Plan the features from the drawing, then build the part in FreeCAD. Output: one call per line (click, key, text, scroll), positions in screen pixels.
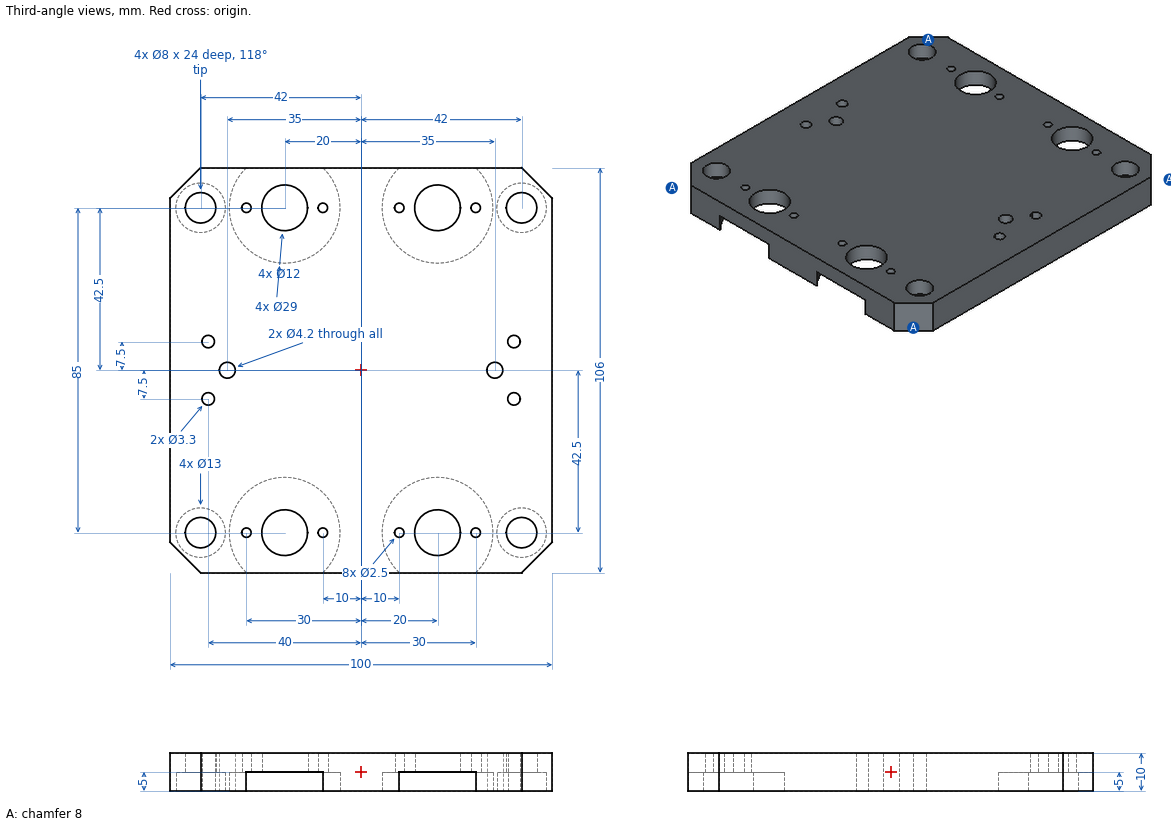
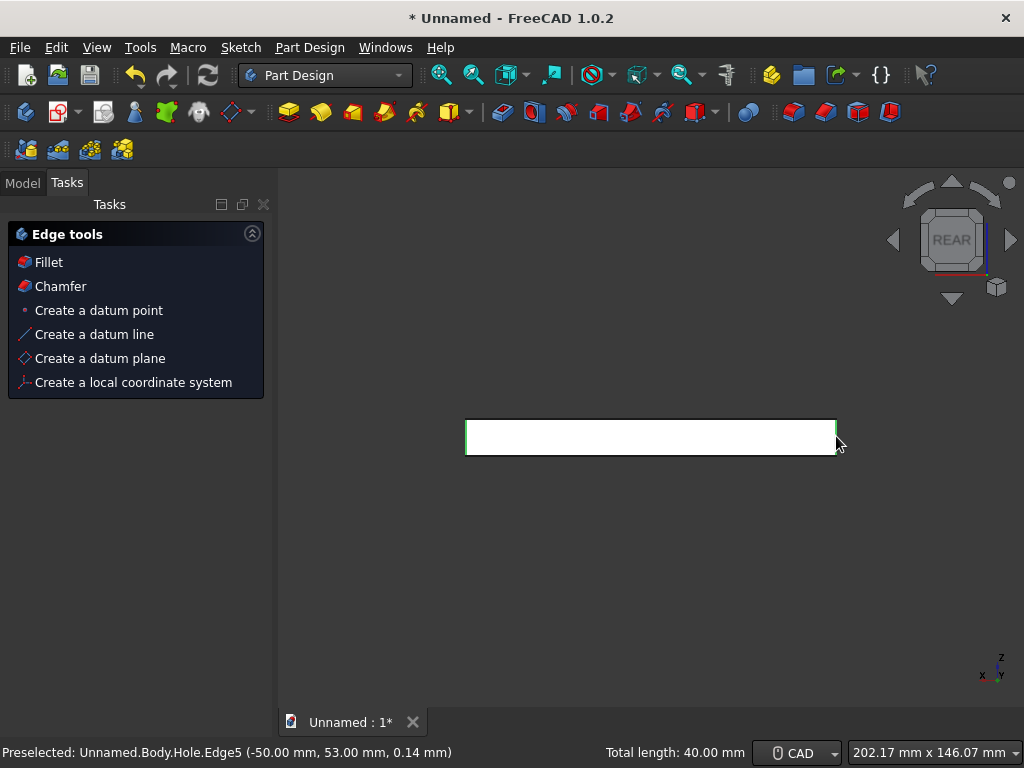
click(826, 112)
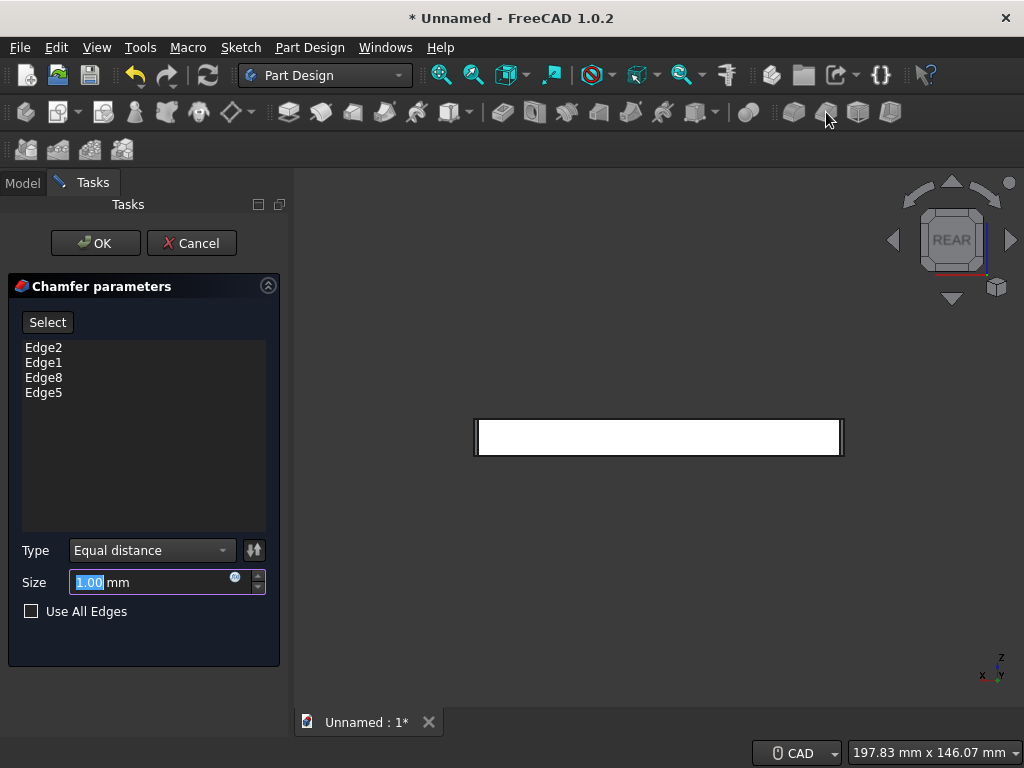
text(8)
key(Tab)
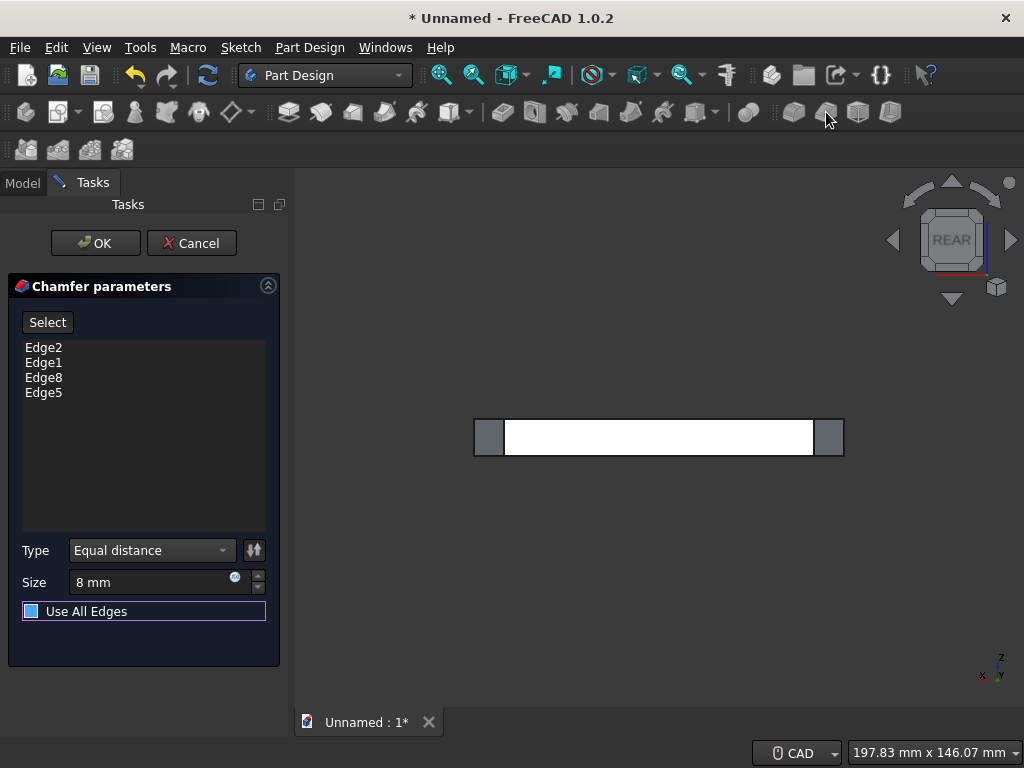
click(96, 243)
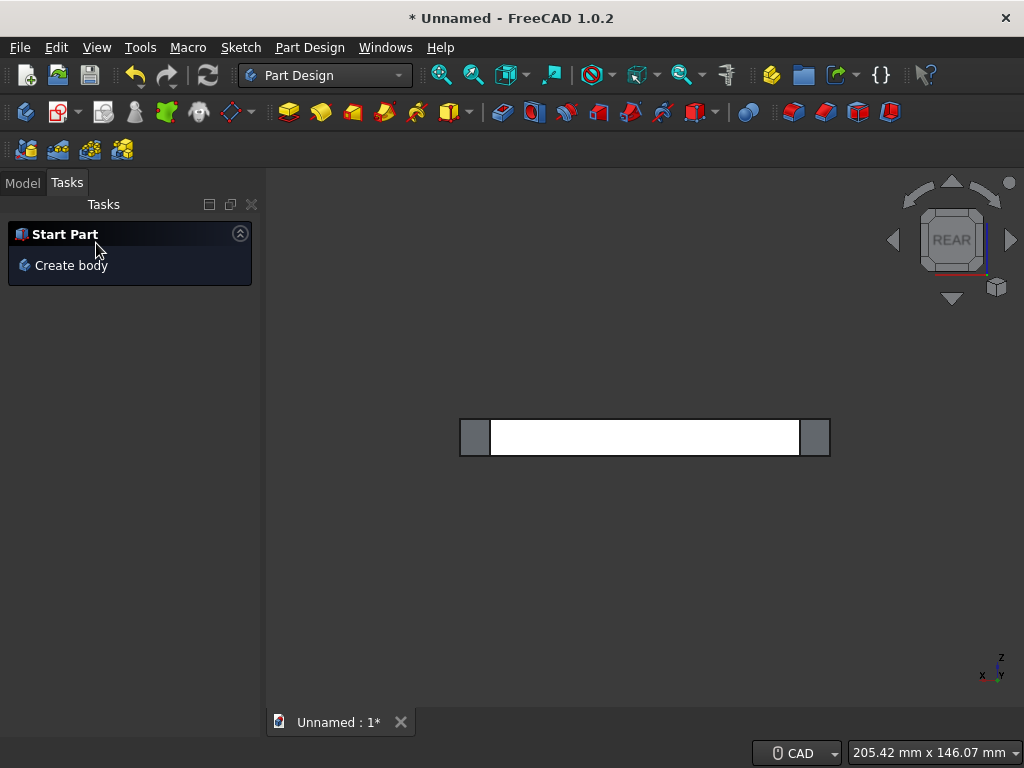
key(0)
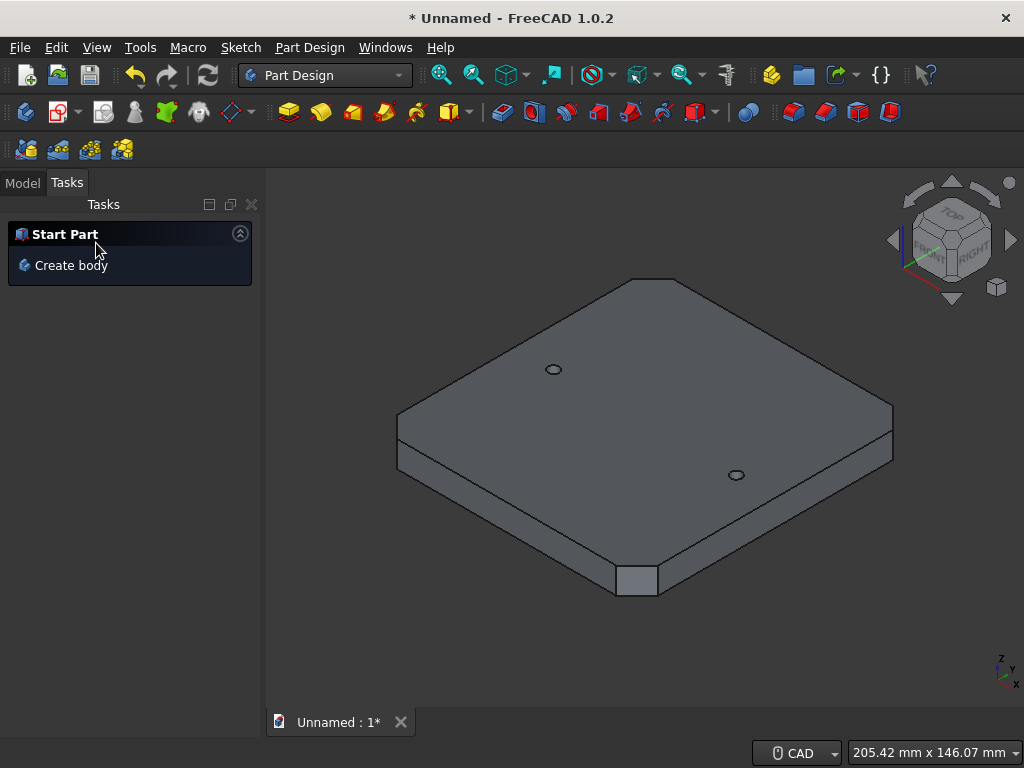
click(685, 399)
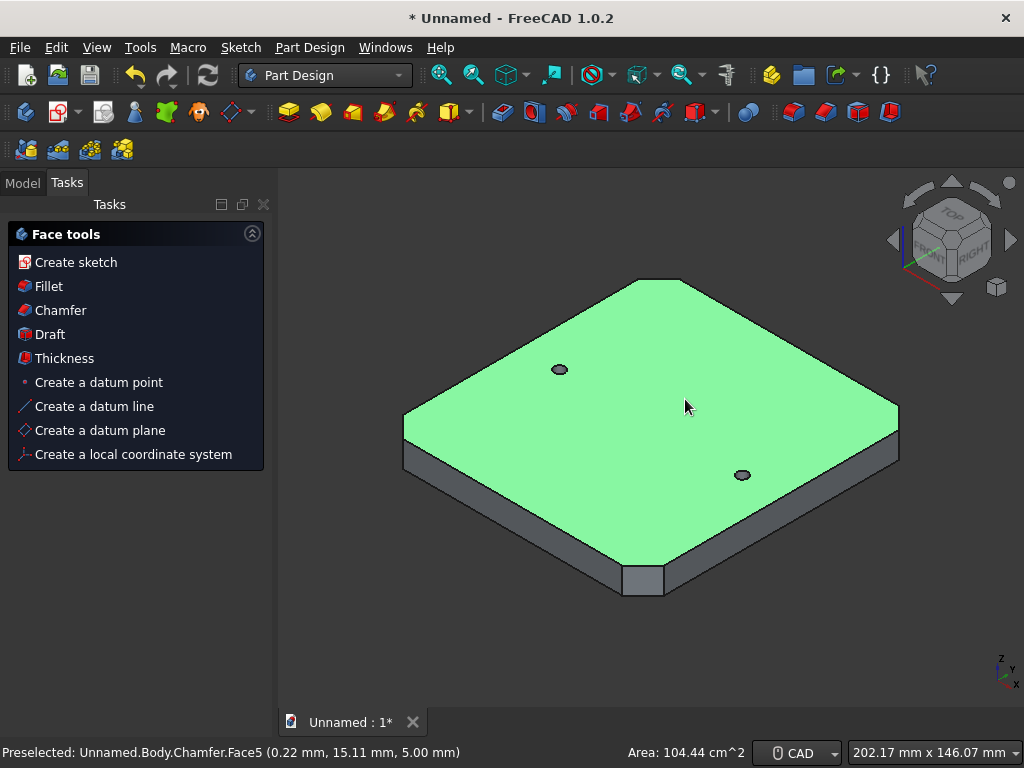
click(58, 112)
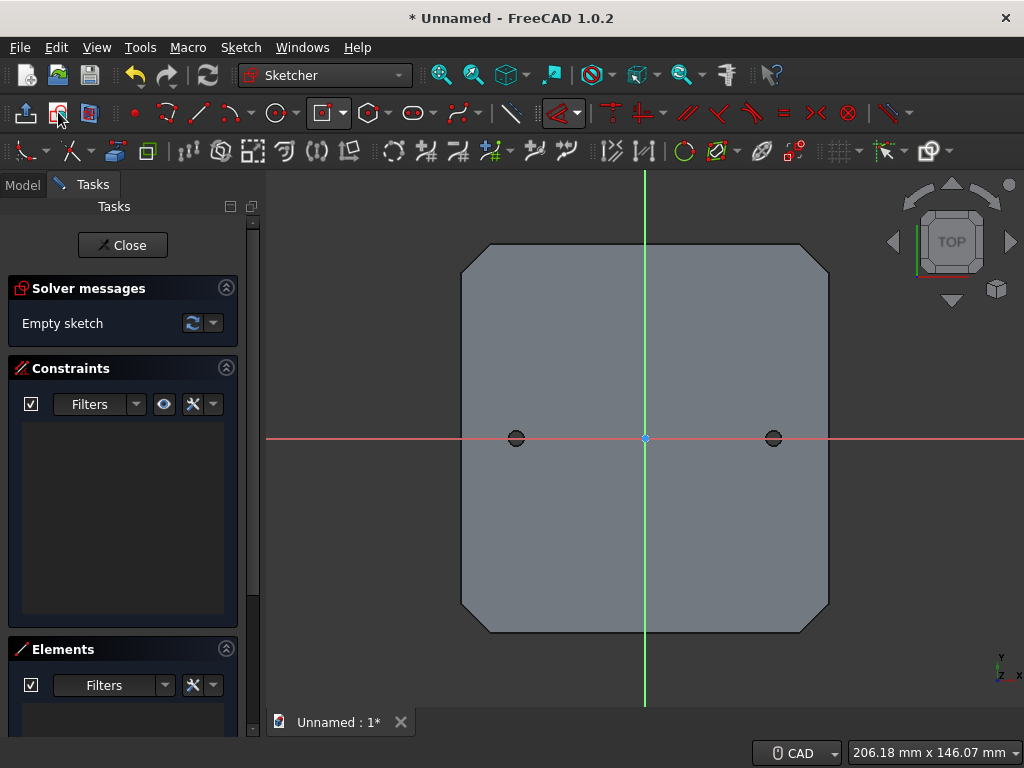
scroll(564, 439, up, 5)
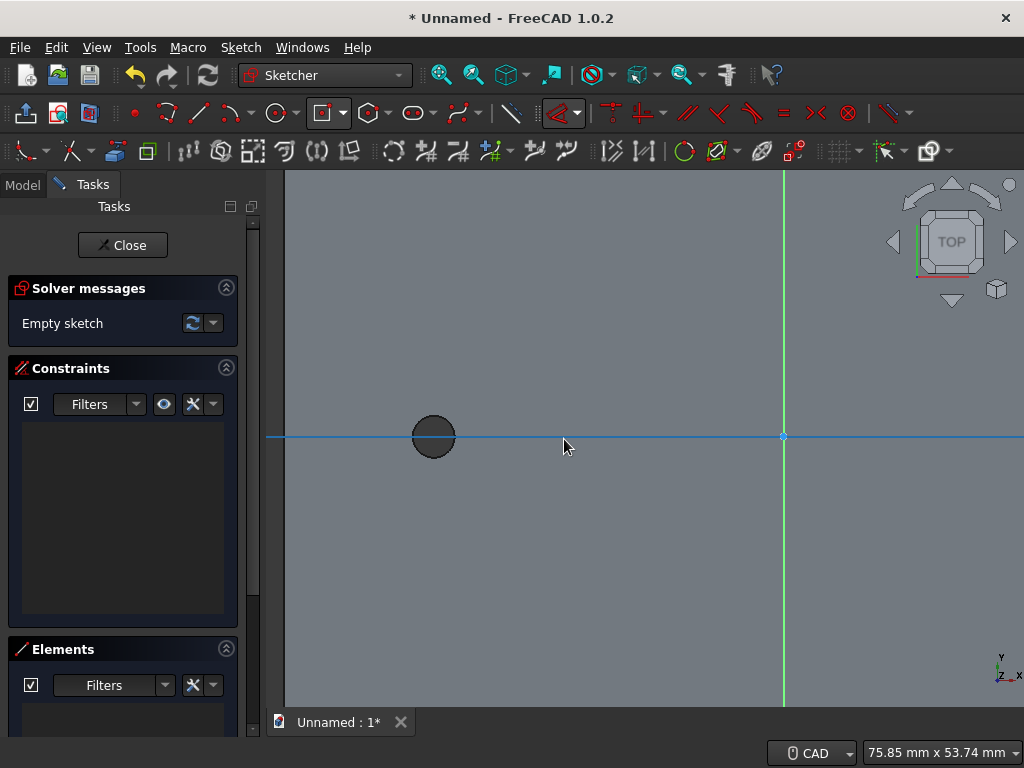
click(276, 114)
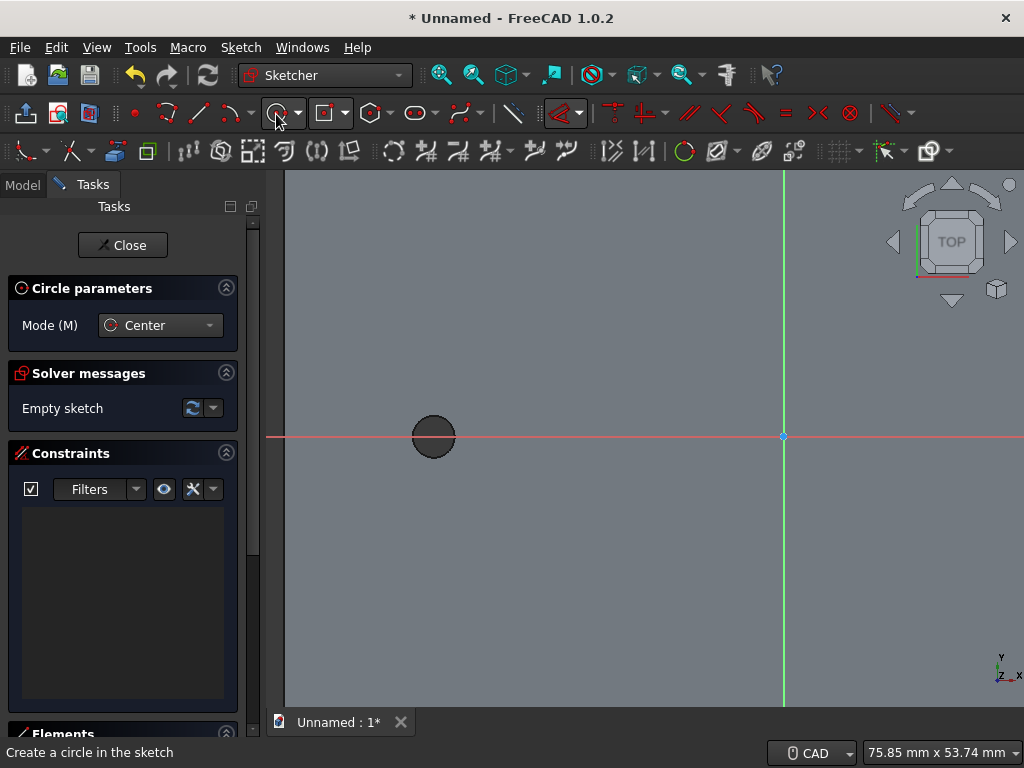
scroll(384, 512, up, 2)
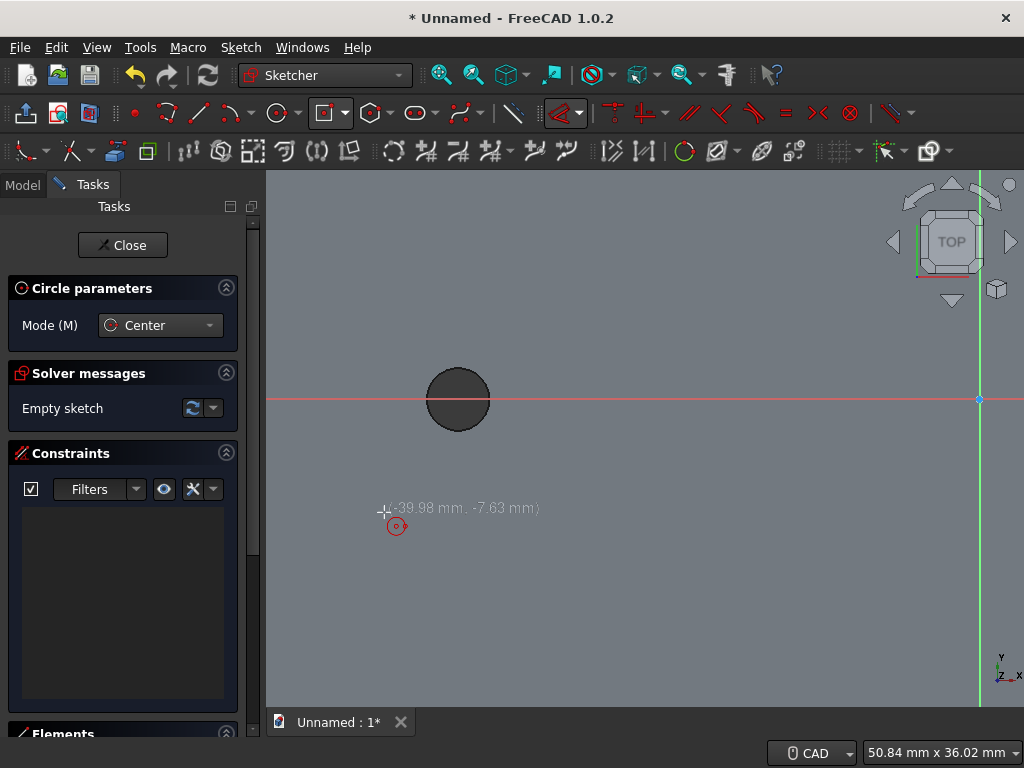
click(384, 511)
move(401, 494)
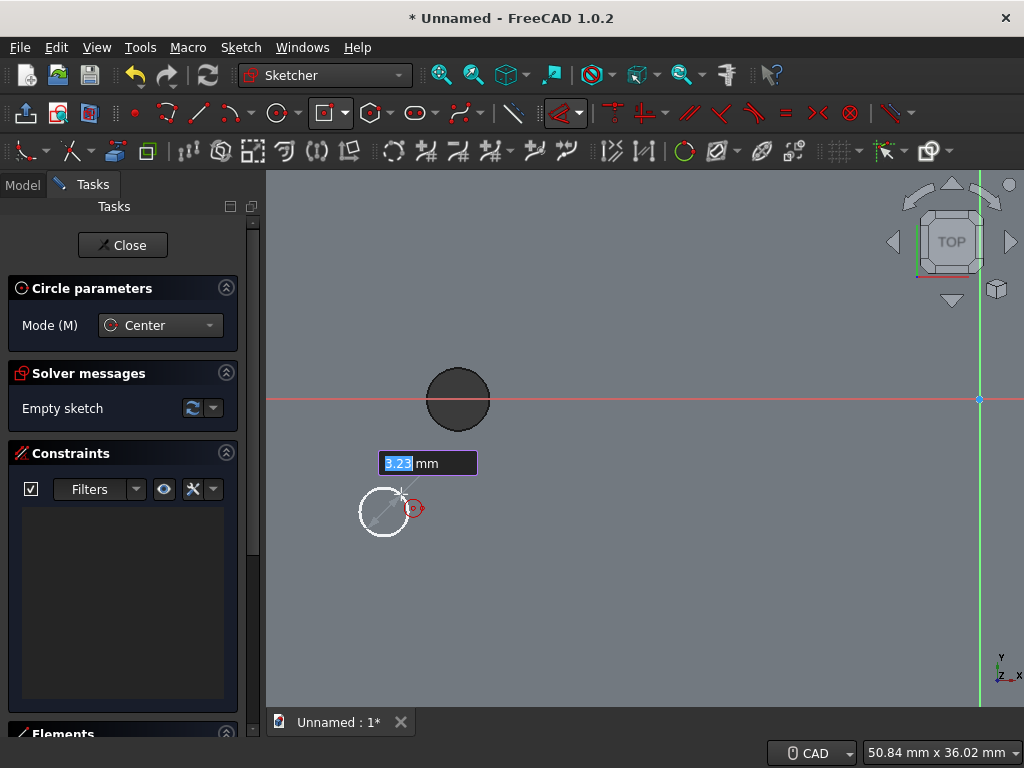
text(3.3)
key(Return)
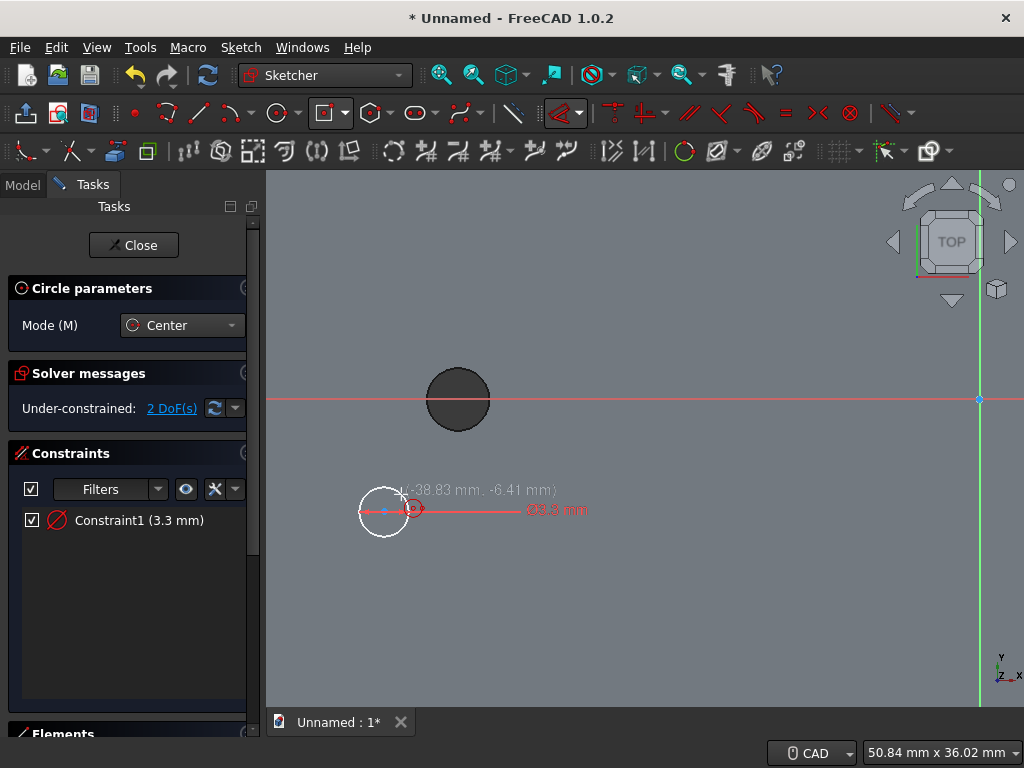
click(384, 288)
move(401, 270)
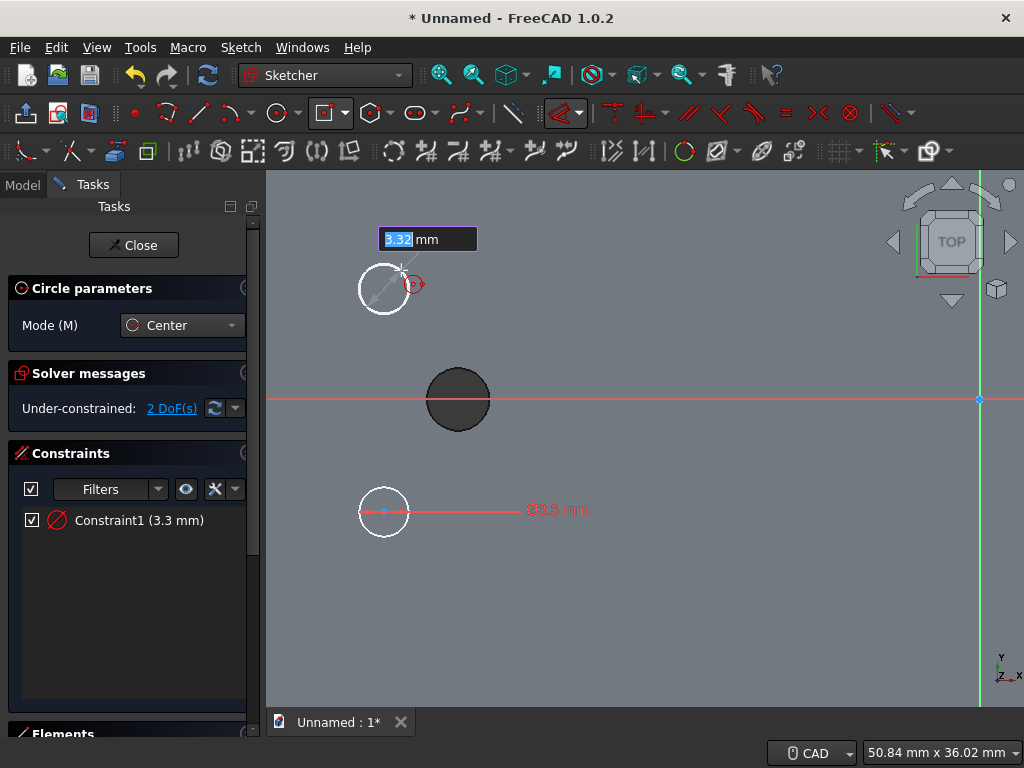
text(3.3)
key(Return)
key(Escape)